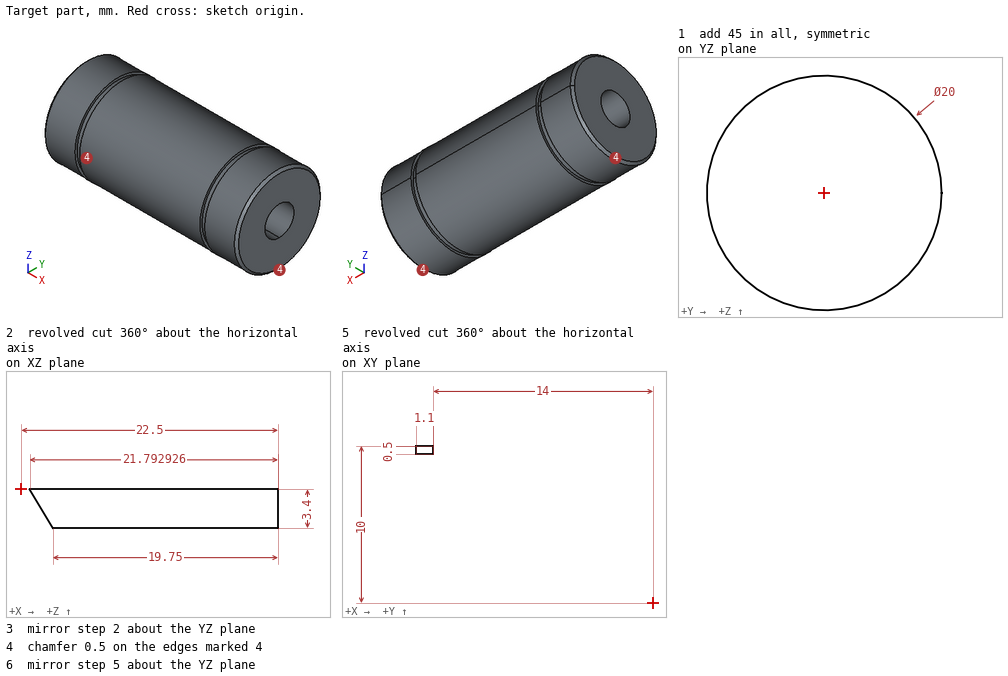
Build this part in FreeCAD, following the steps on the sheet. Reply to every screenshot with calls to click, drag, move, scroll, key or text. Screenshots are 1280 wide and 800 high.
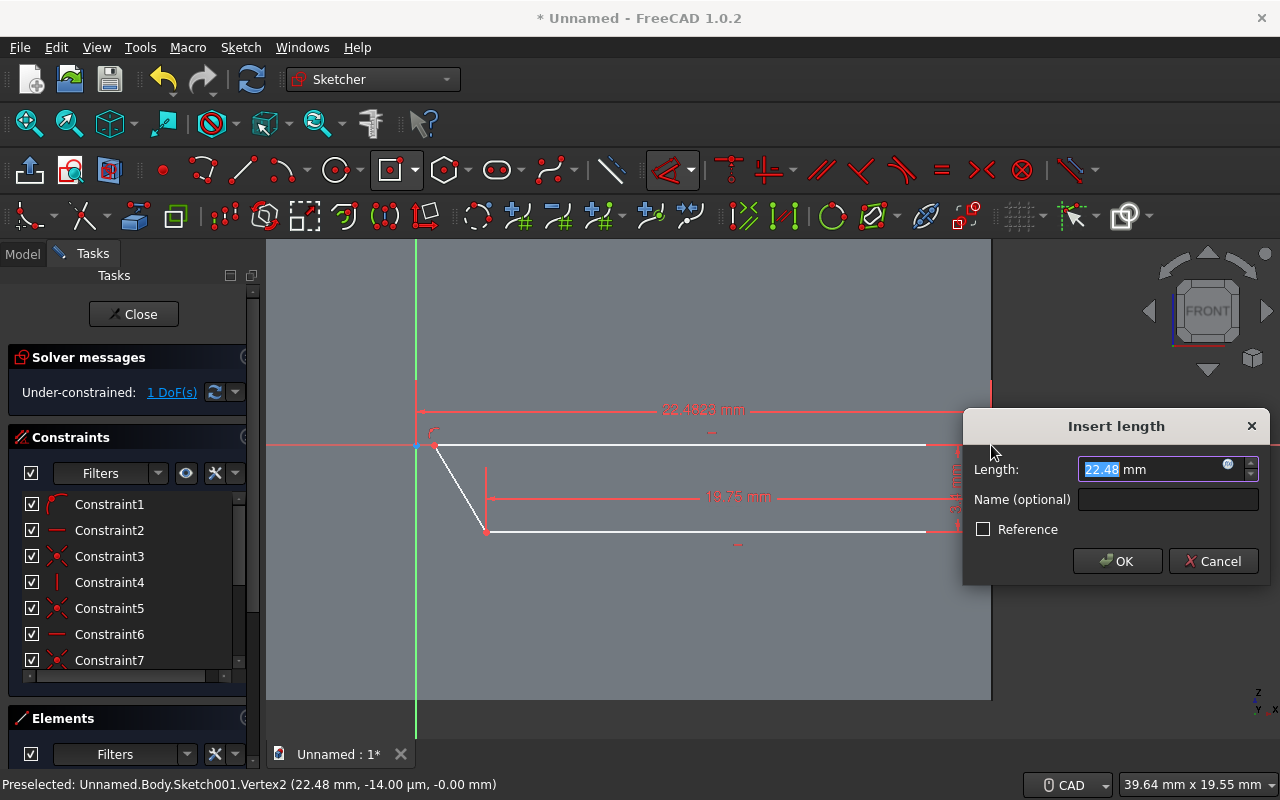
text(22.5)
key(Return)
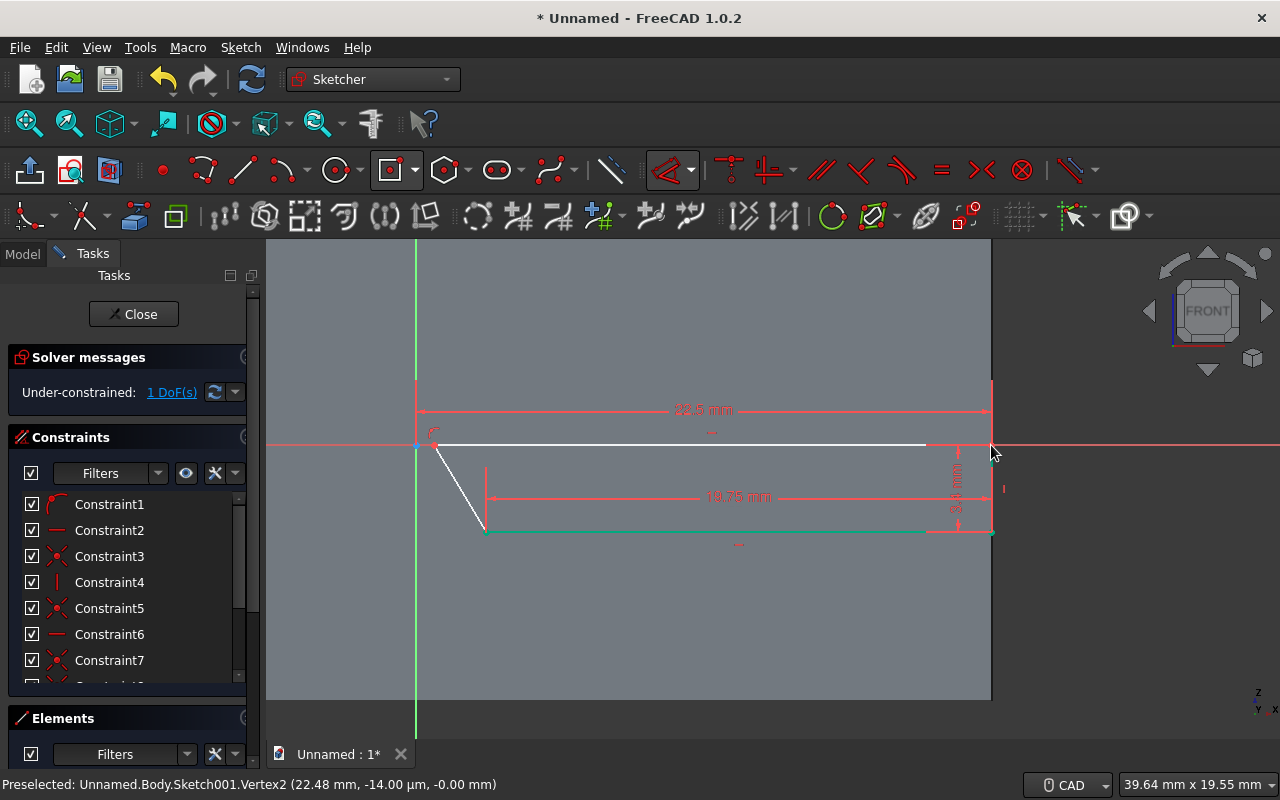
click(601, 445)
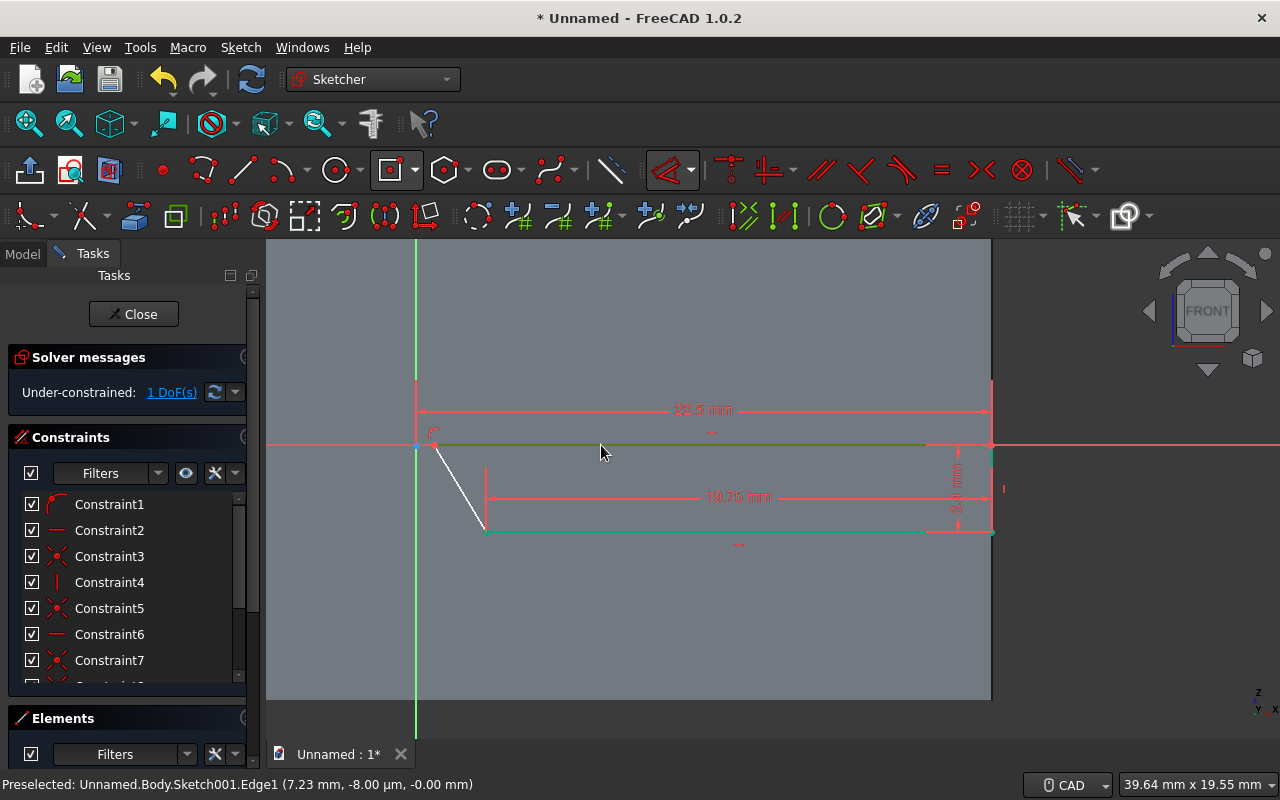
click(694, 170)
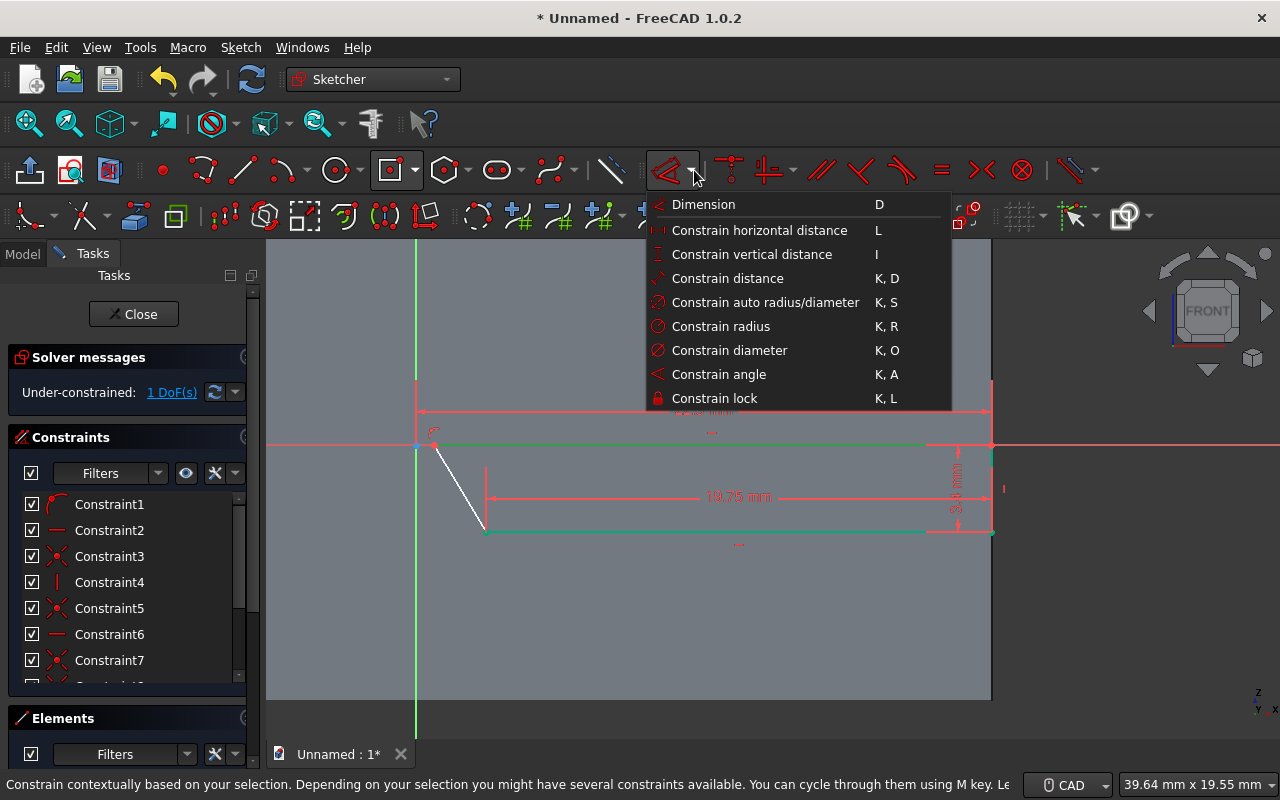
click(799, 230)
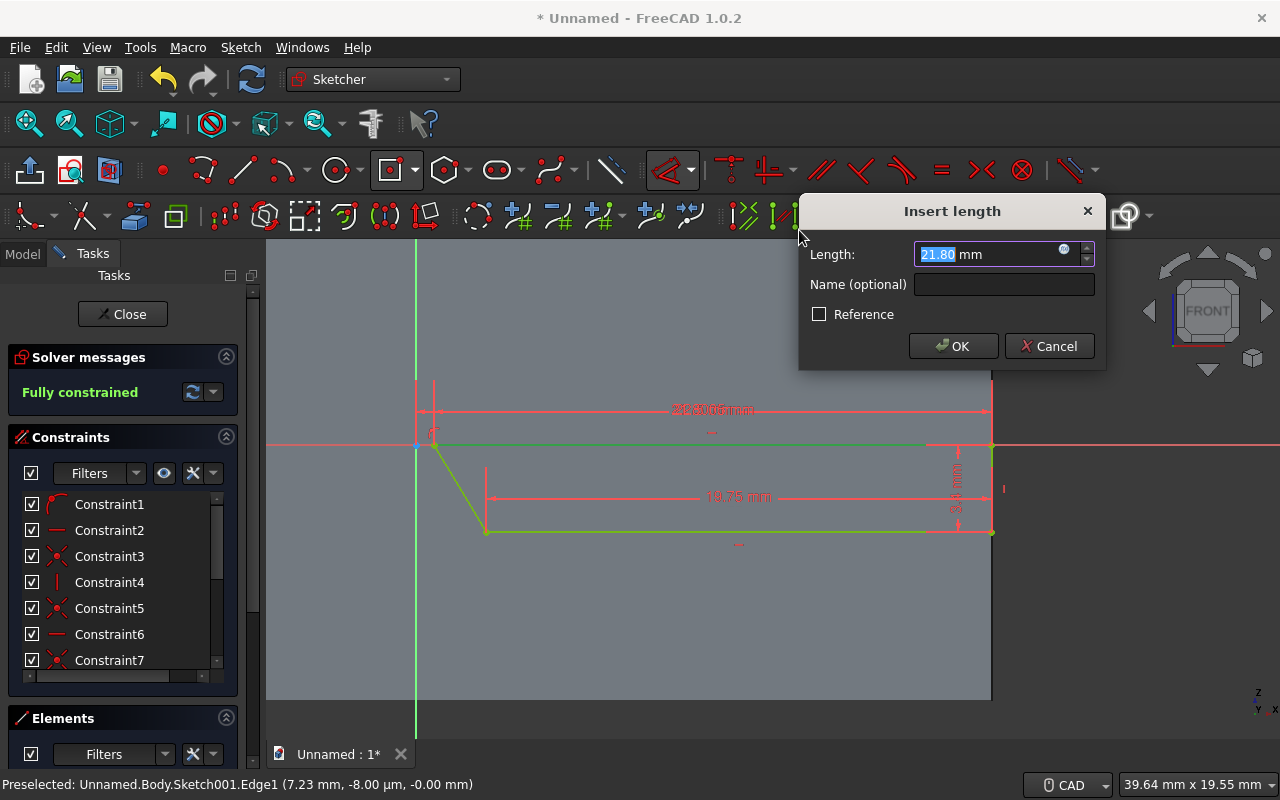
text(21.792926)
key(Return)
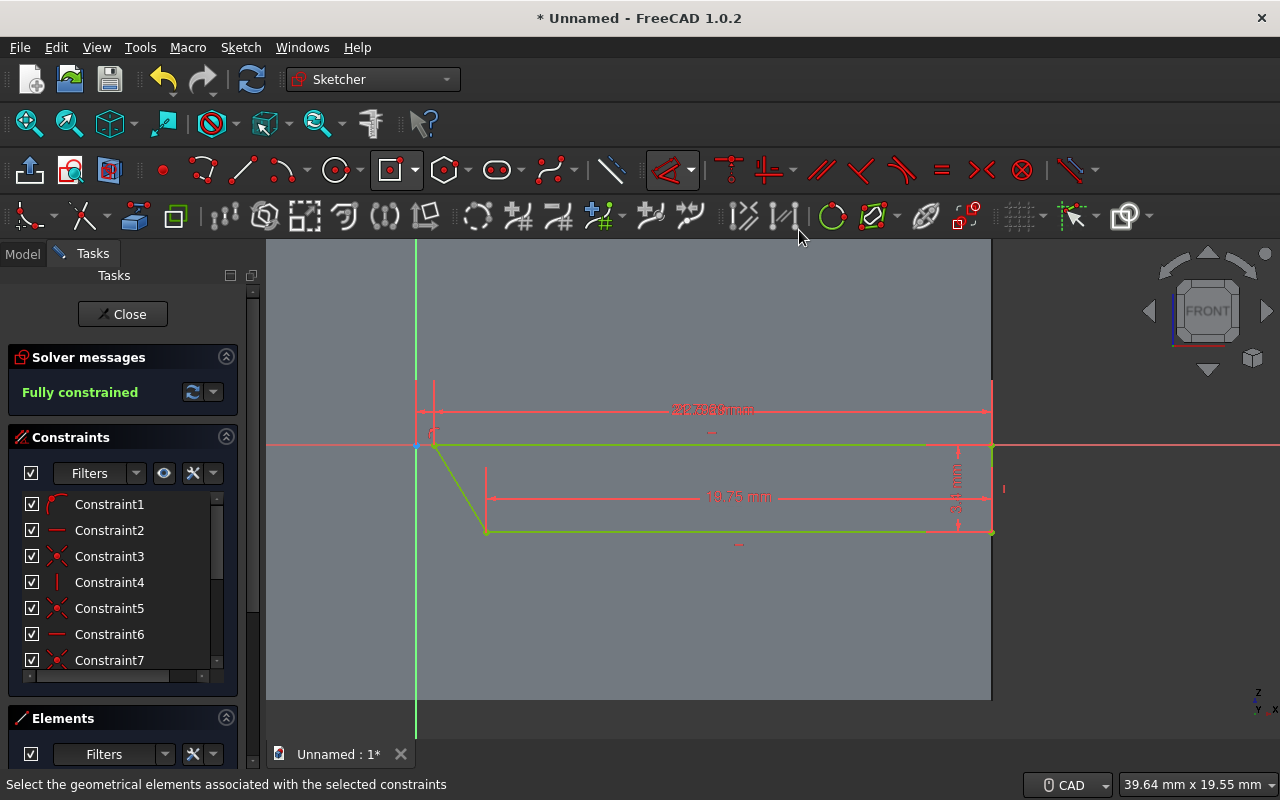
click(123, 314)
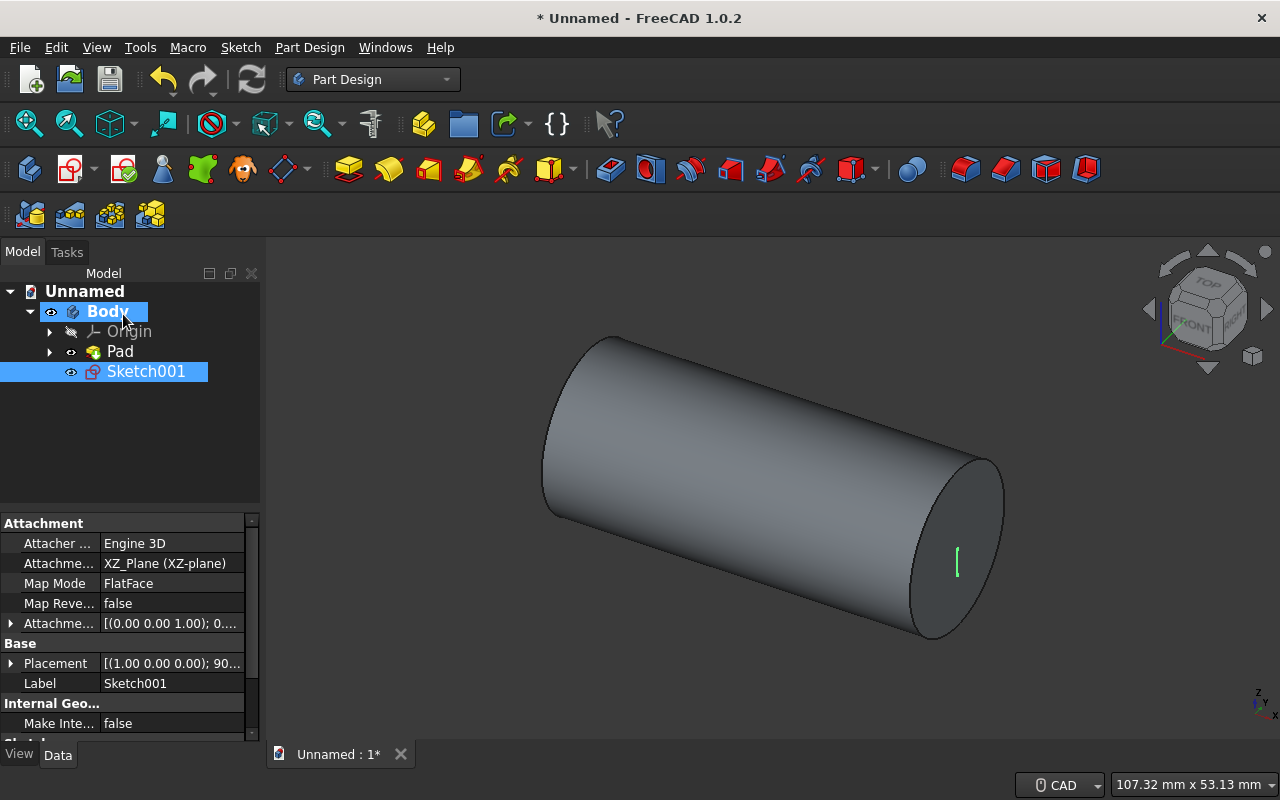
click(692, 170)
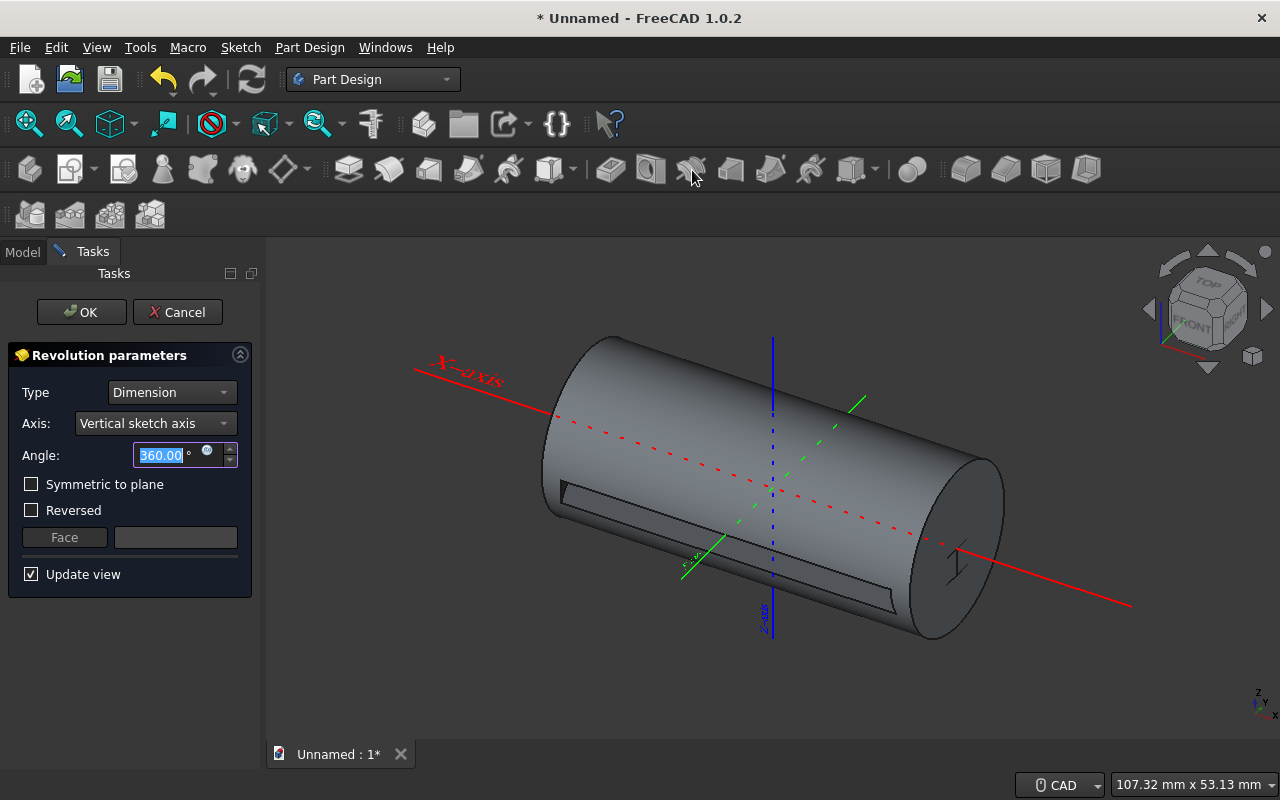
click(156, 424)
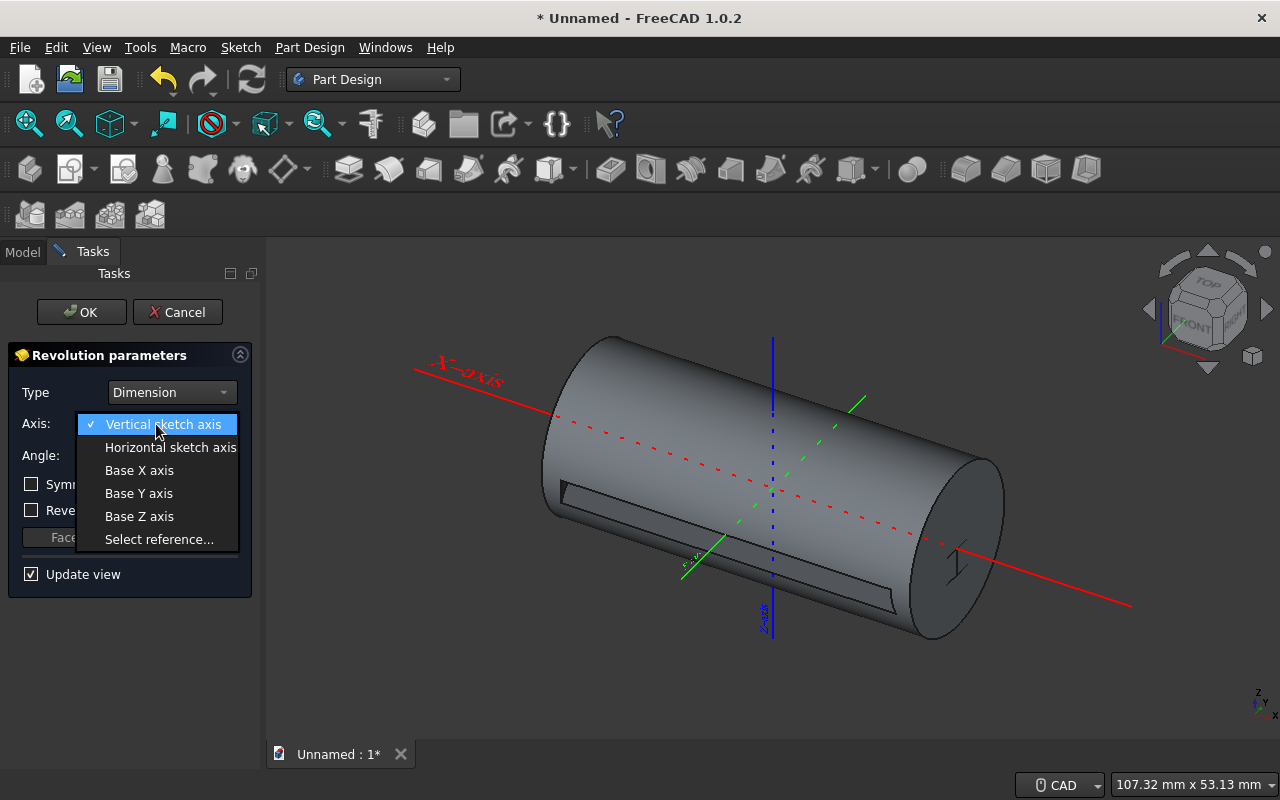
click(156, 448)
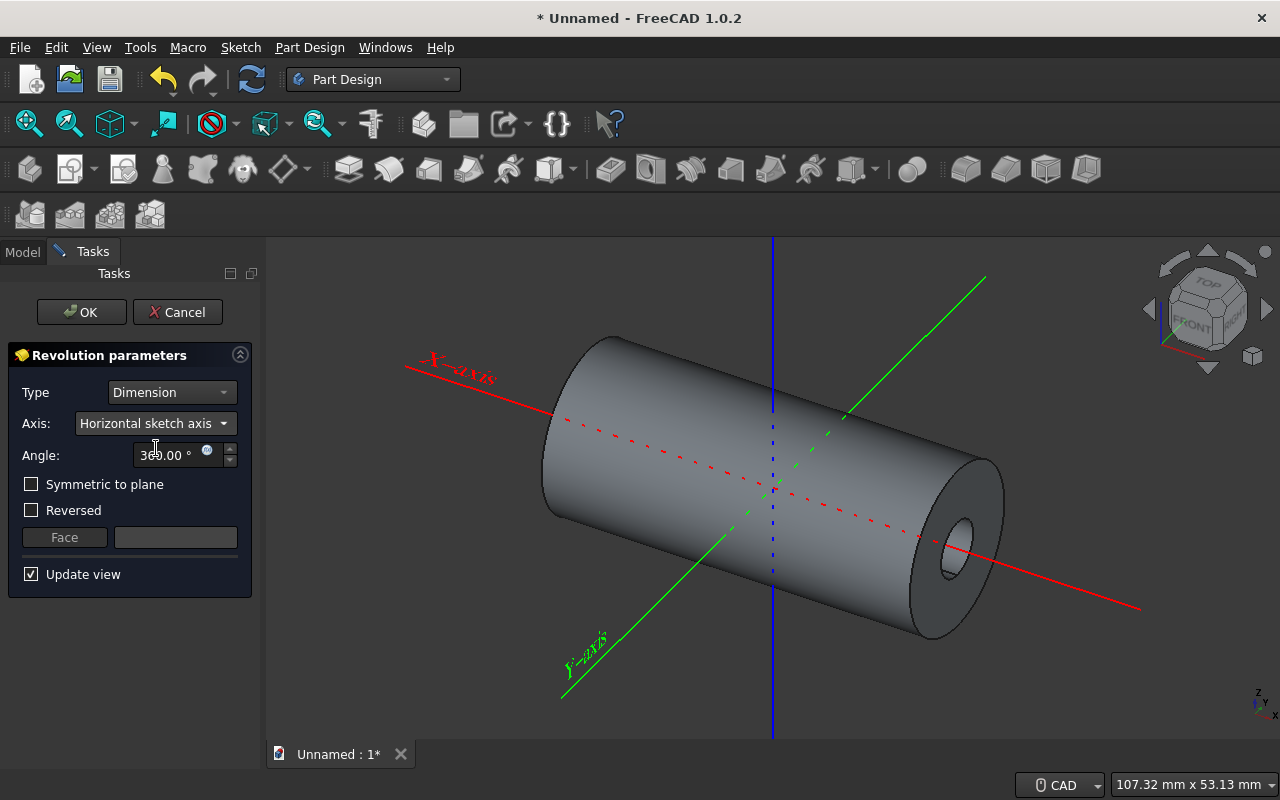
click(82, 312)